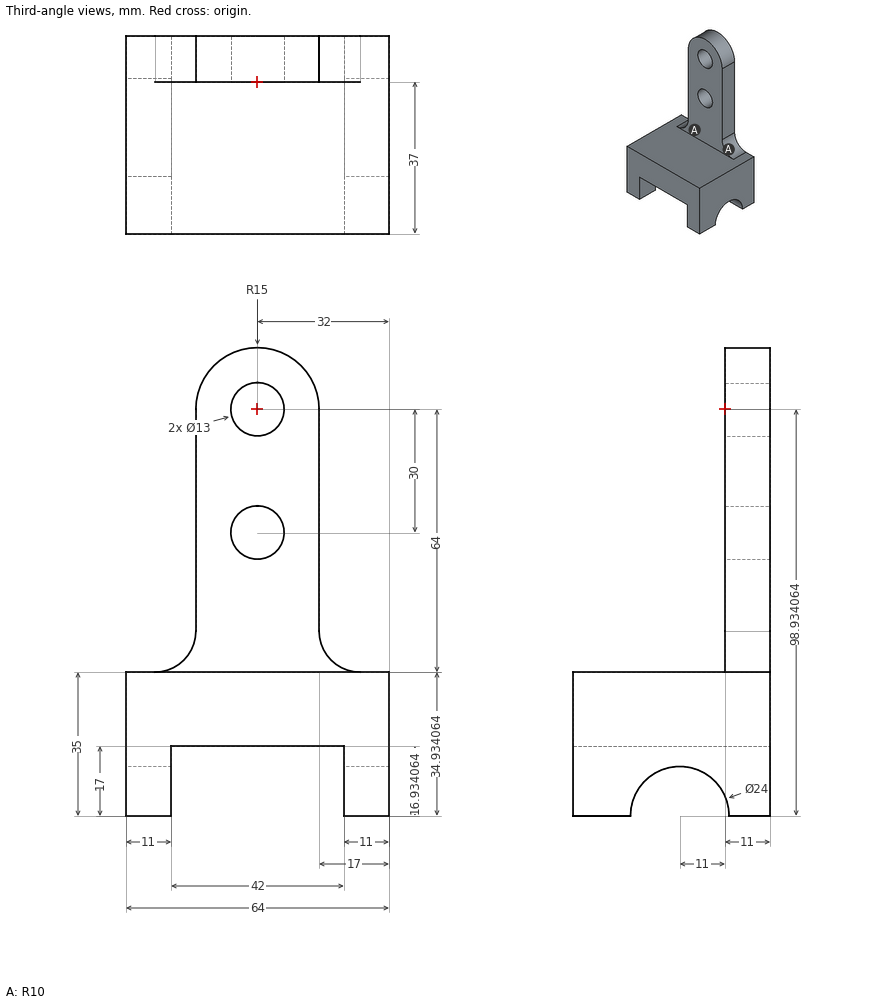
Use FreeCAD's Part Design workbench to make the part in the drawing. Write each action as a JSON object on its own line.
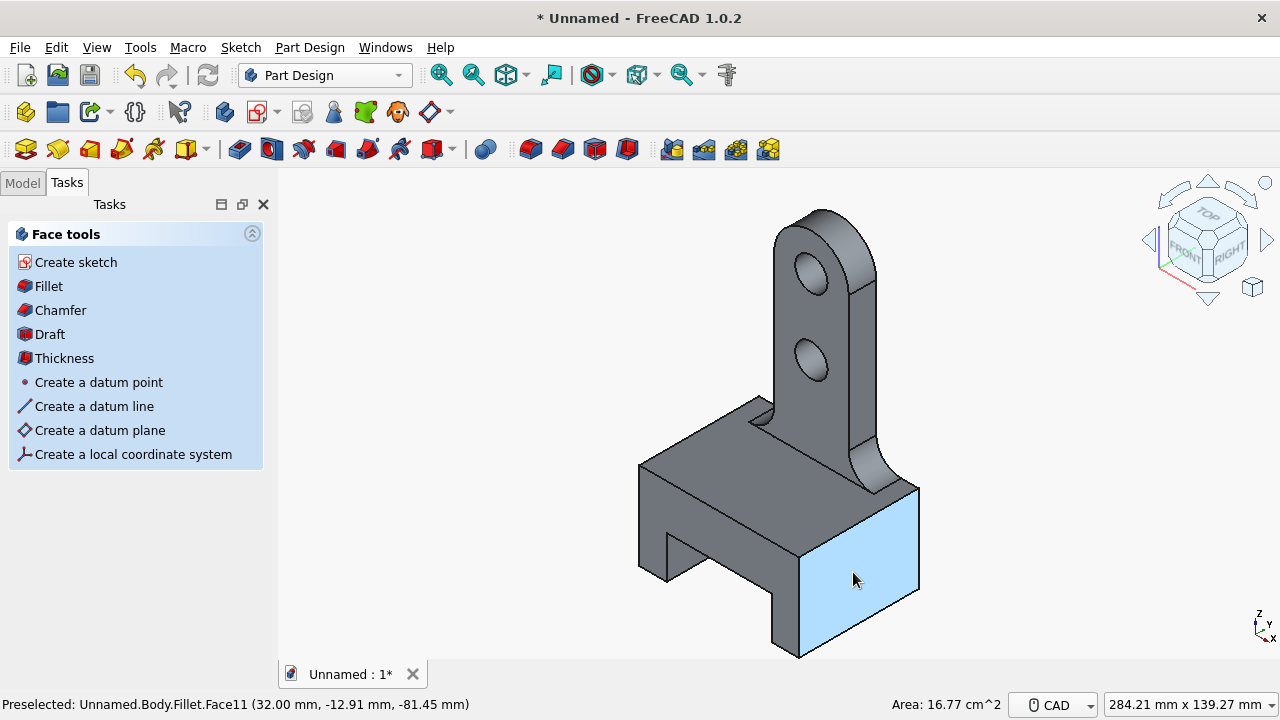
{"action": "left_click", "coordinate": [258, 112]}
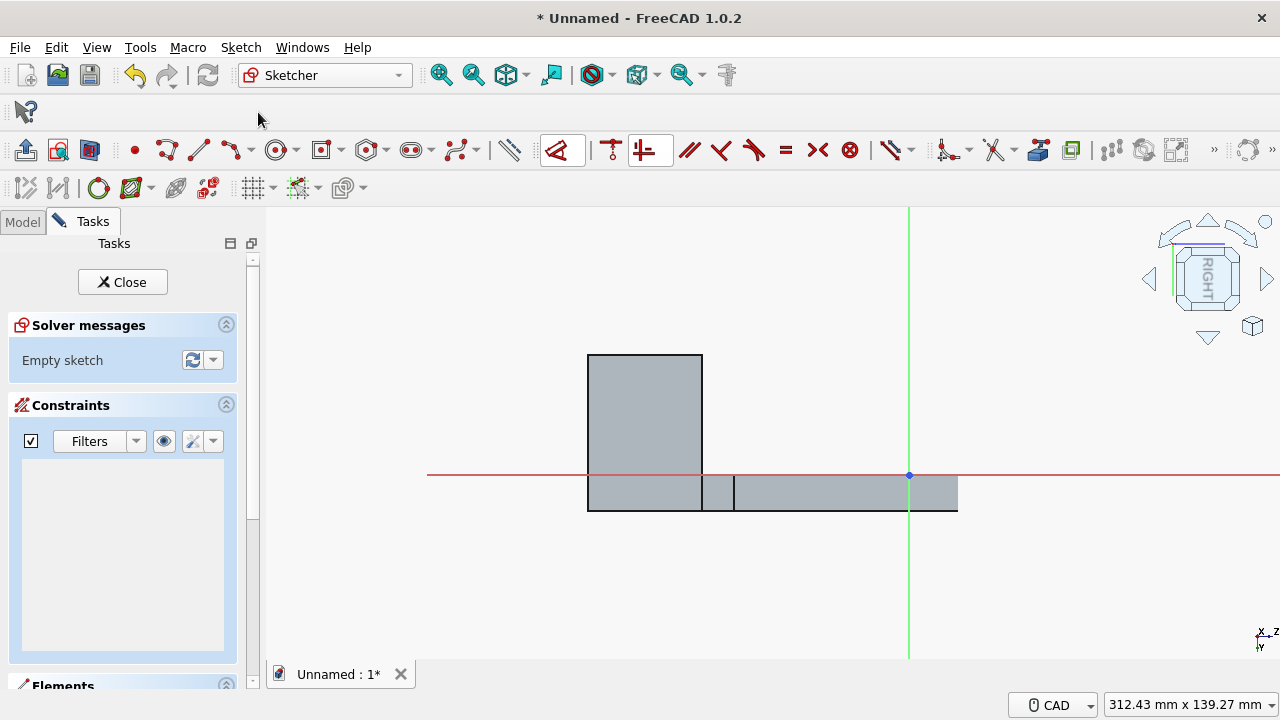
{"action": "scroll", "coordinate": [538, 442], "scroll_direction": "up", "scroll_amount": 6}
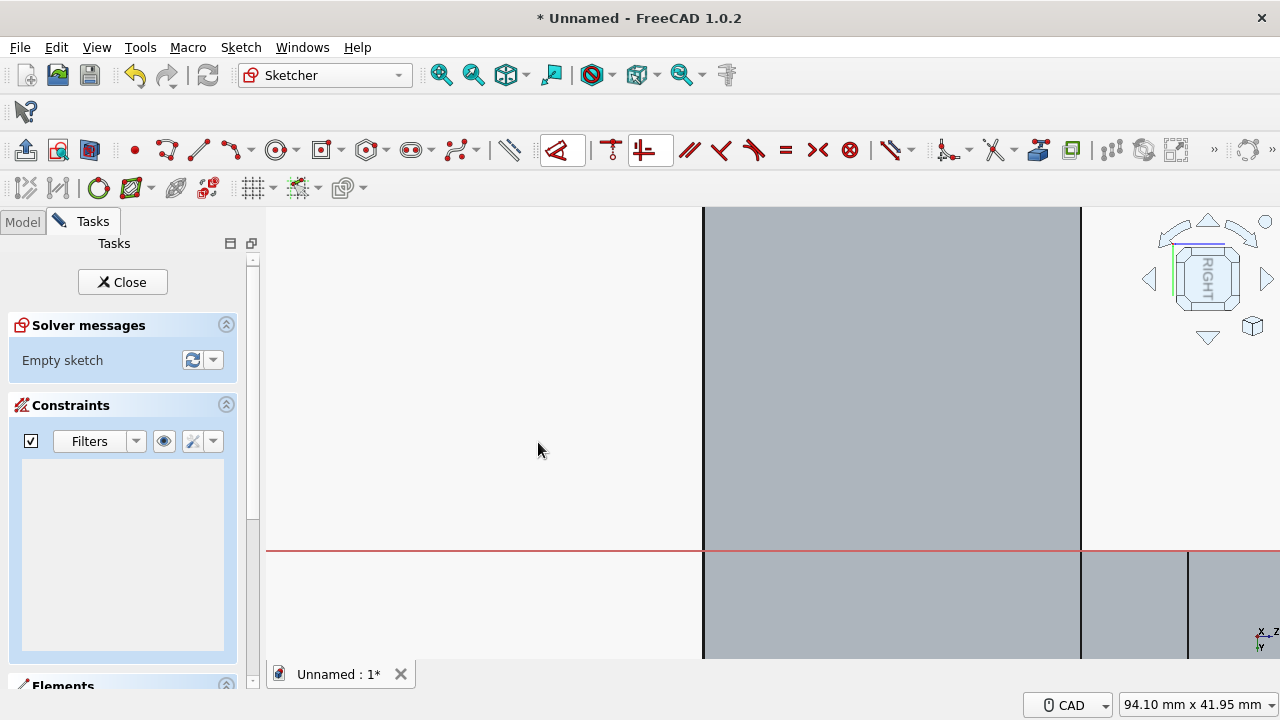
{"action": "left_click", "coordinate": [276, 150]}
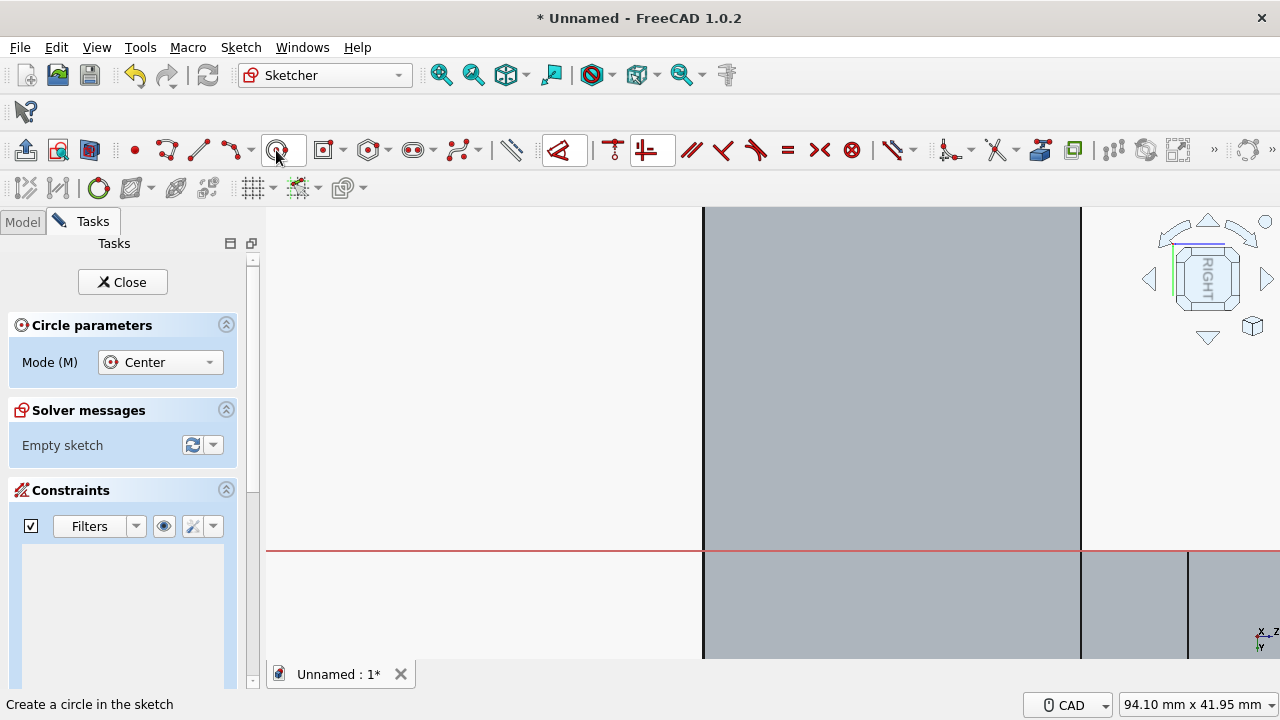
{"action": "left_click", "coordinate": [704, 432]}
{"action": "left_click", "coordinate": [796, 341]}
{"action": "key", "text": "Escape"}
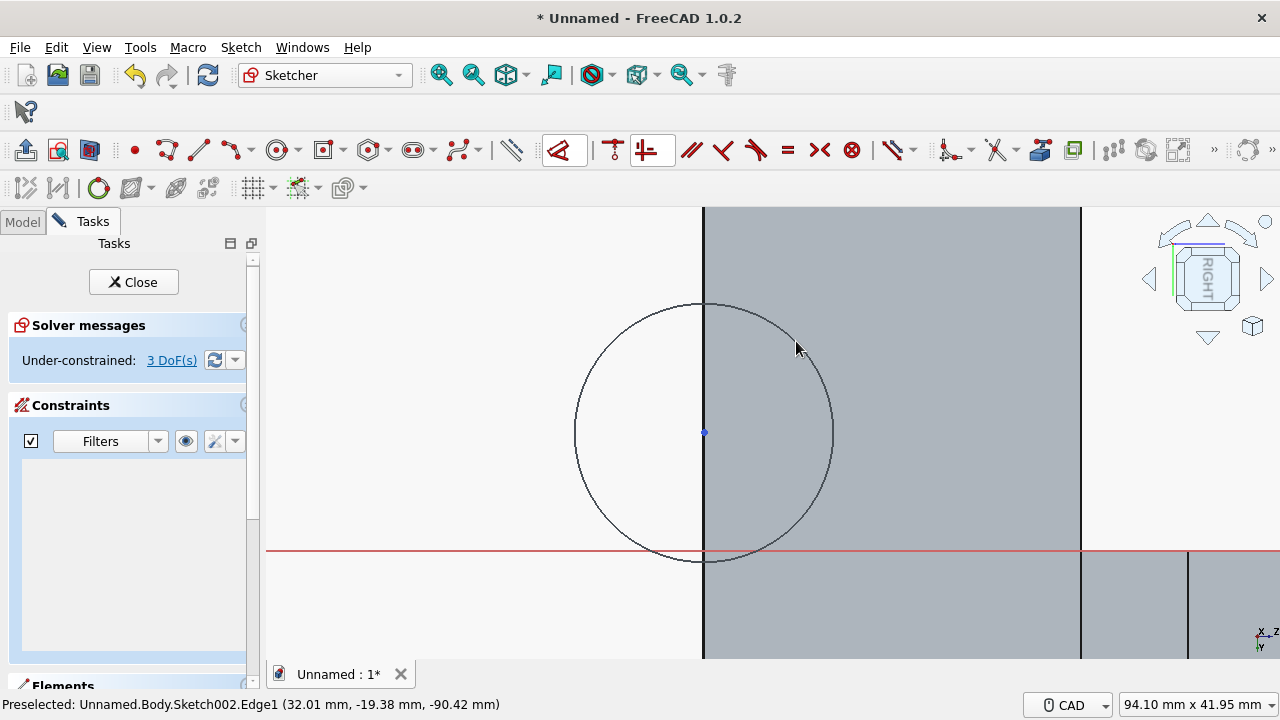
{"action": "left_click", "coordinate": [795, 341]}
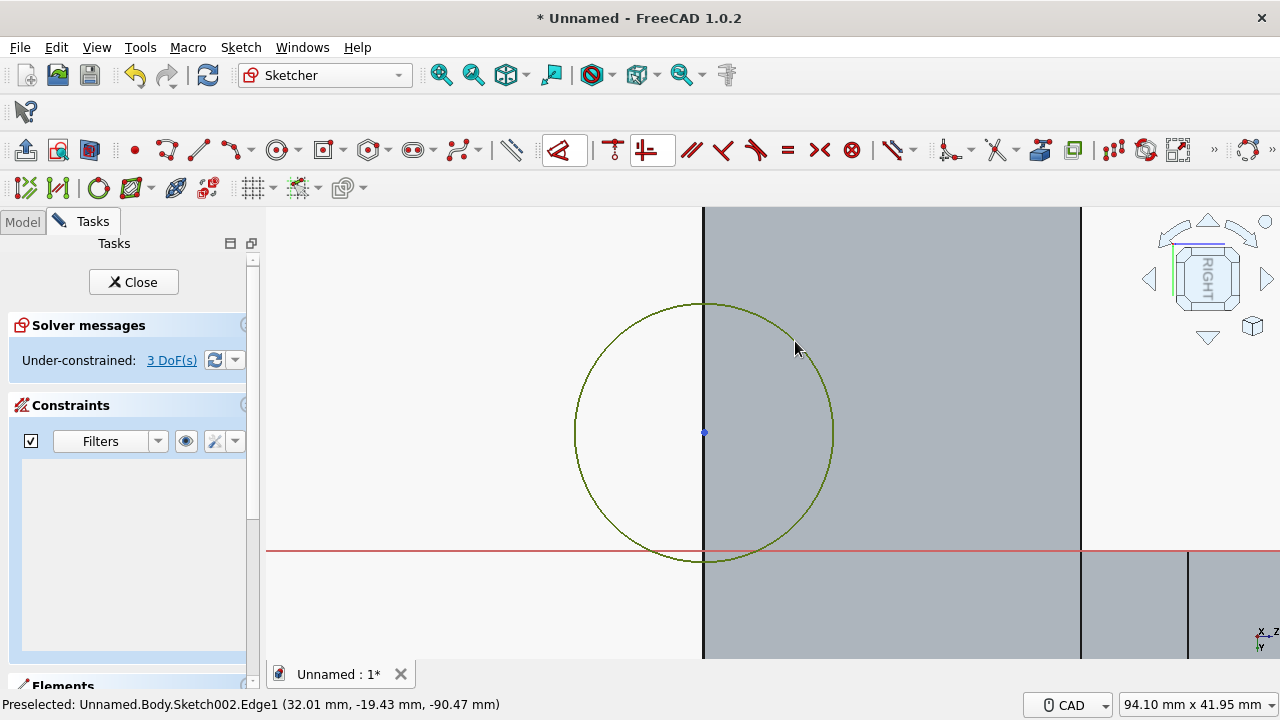
{"action": "left_click", "coordinate": [582, 150]}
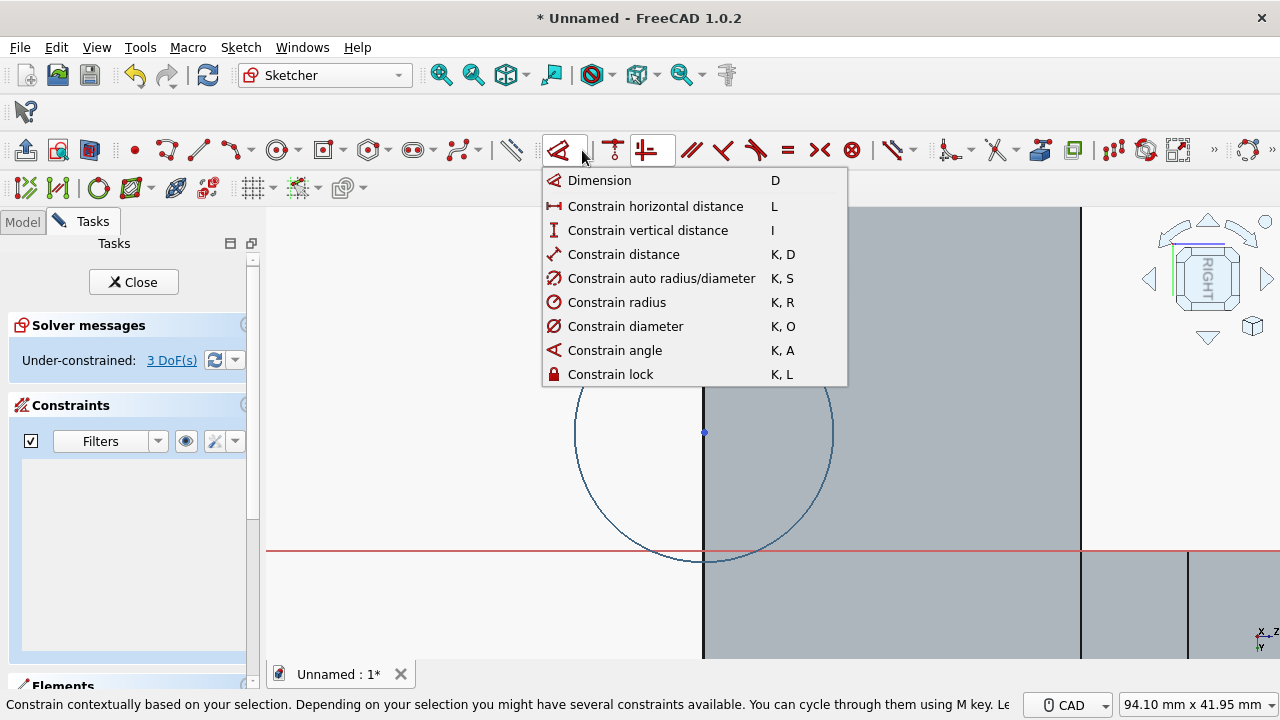
{"action": "left_click", "coordinate": [695, 326]}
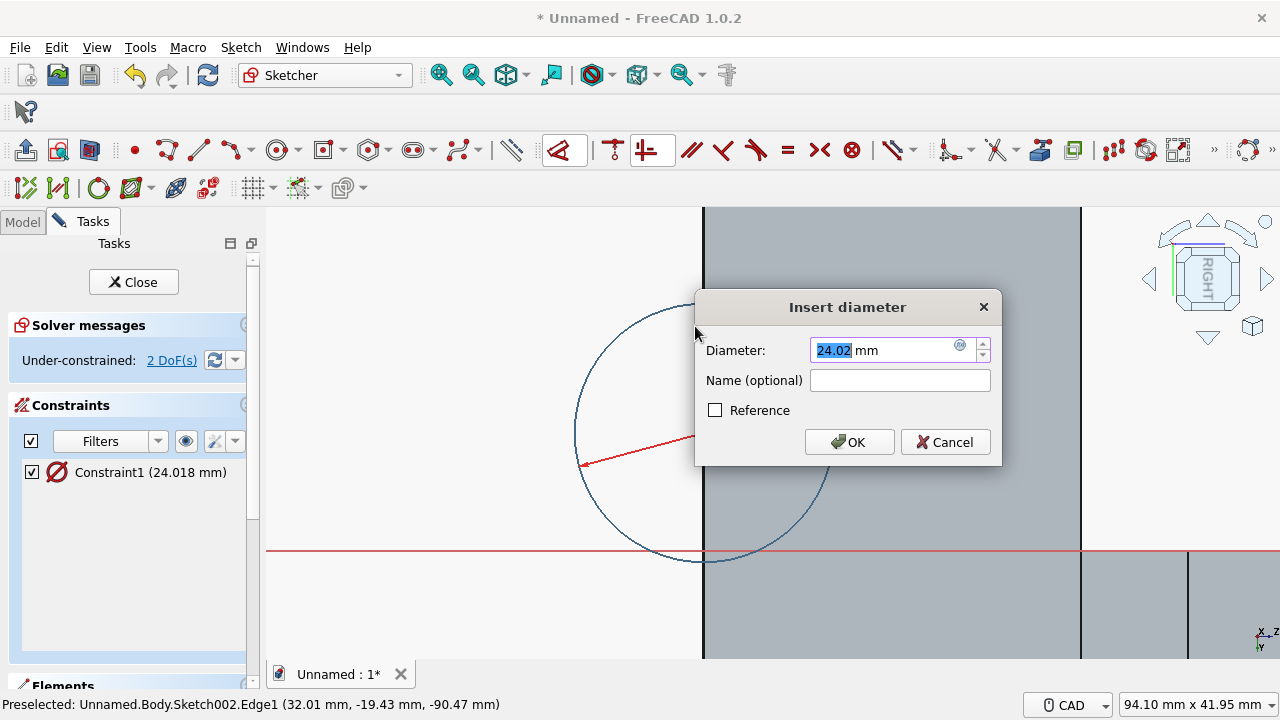
{"action": "type", "text": "24"}
{"action": "key", "text": "Return"}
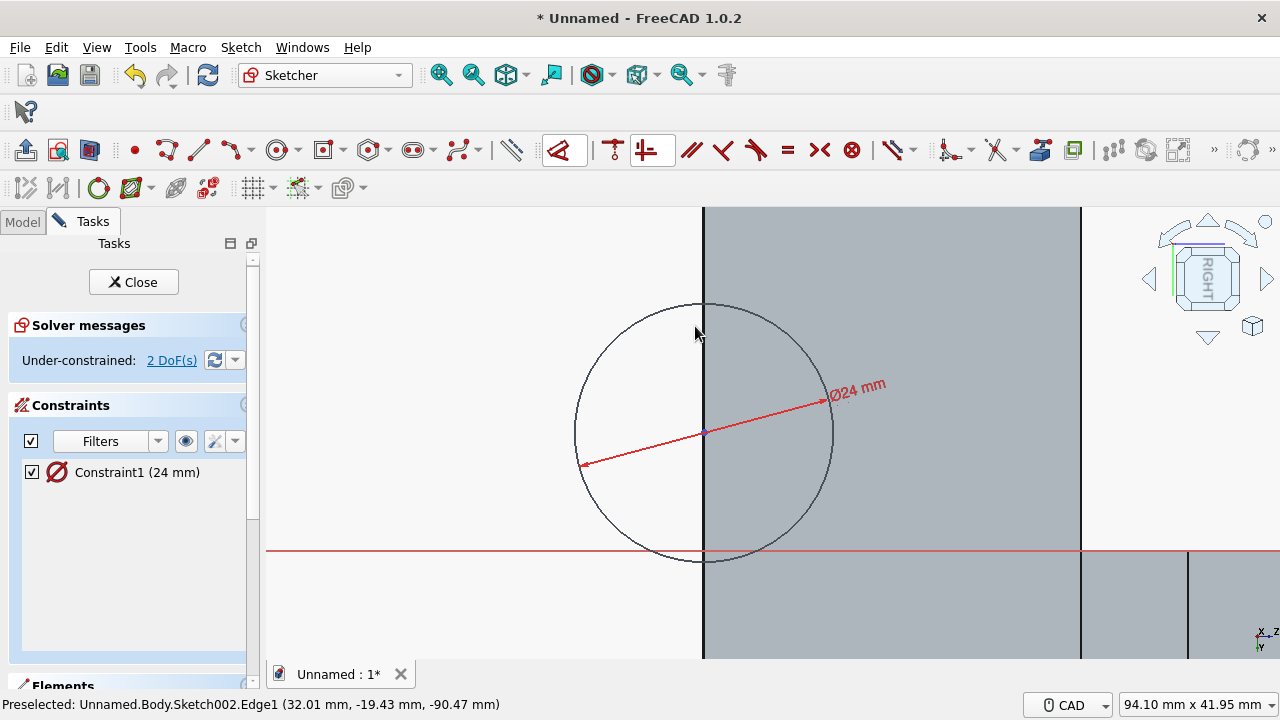
{"action": "left_click", "coordinate": [704, 433]}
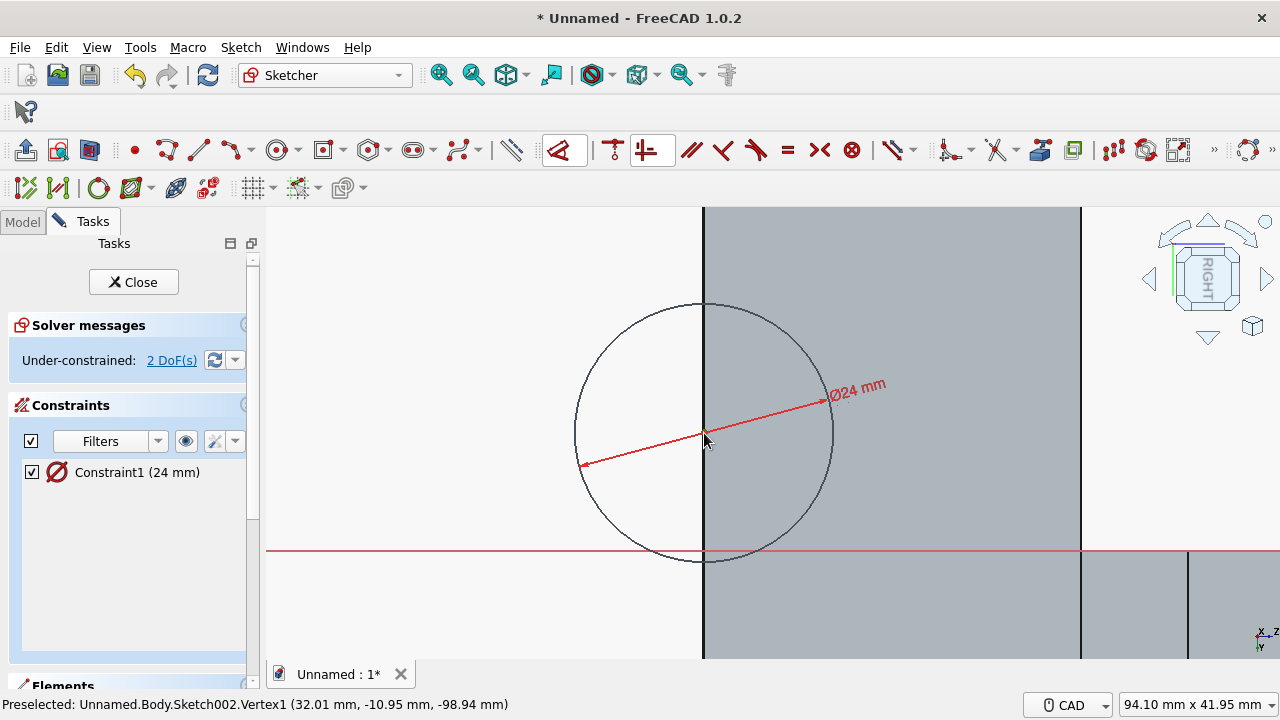
{"action": "left_click", "coordinate": [582, 150]}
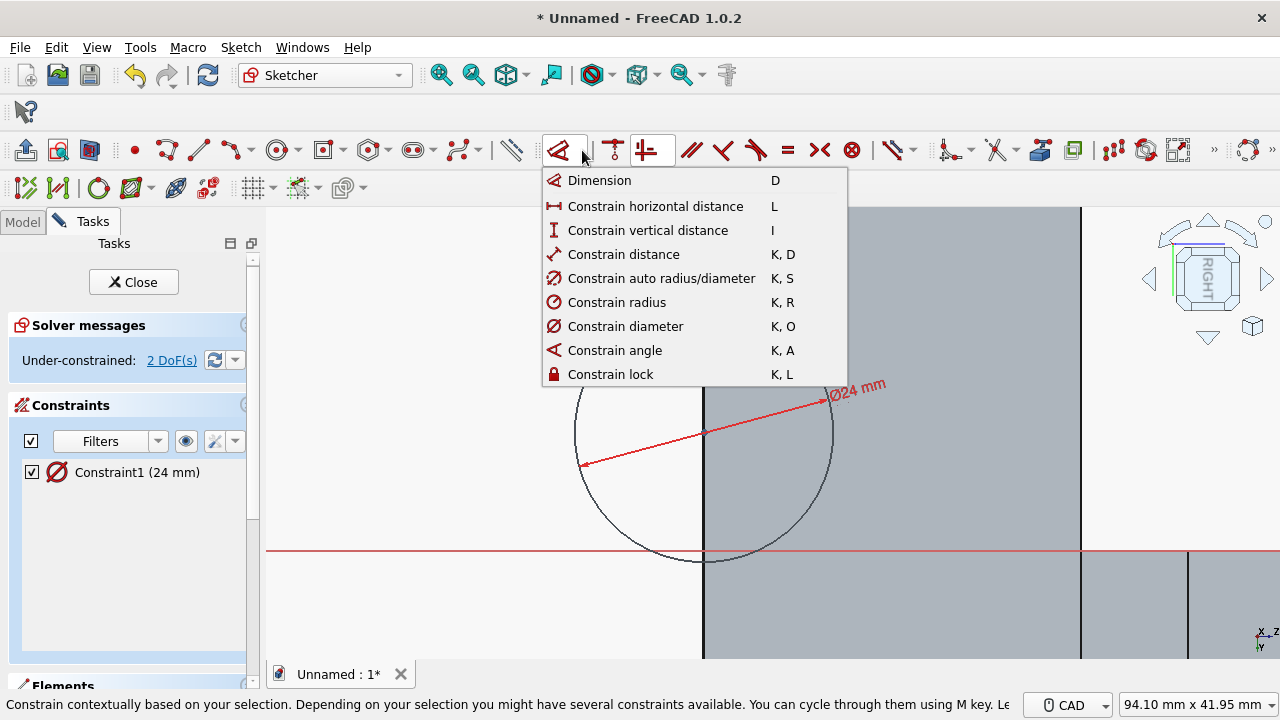
{"action": "left_click", "coordinate": [695, 230]}